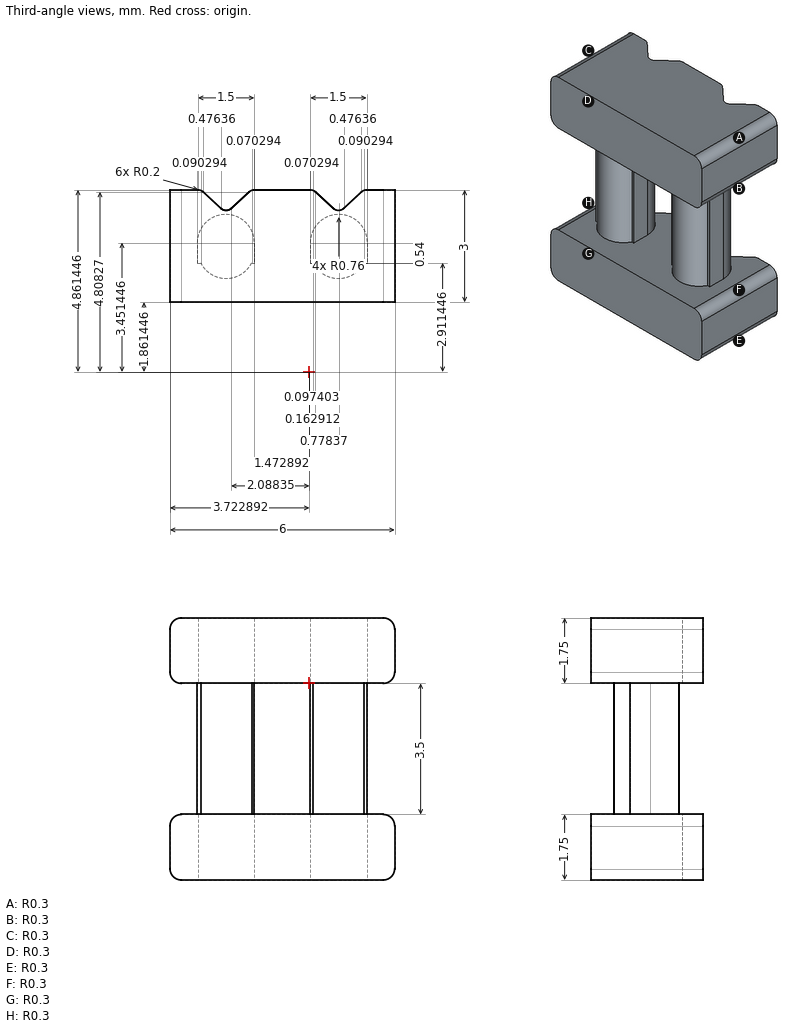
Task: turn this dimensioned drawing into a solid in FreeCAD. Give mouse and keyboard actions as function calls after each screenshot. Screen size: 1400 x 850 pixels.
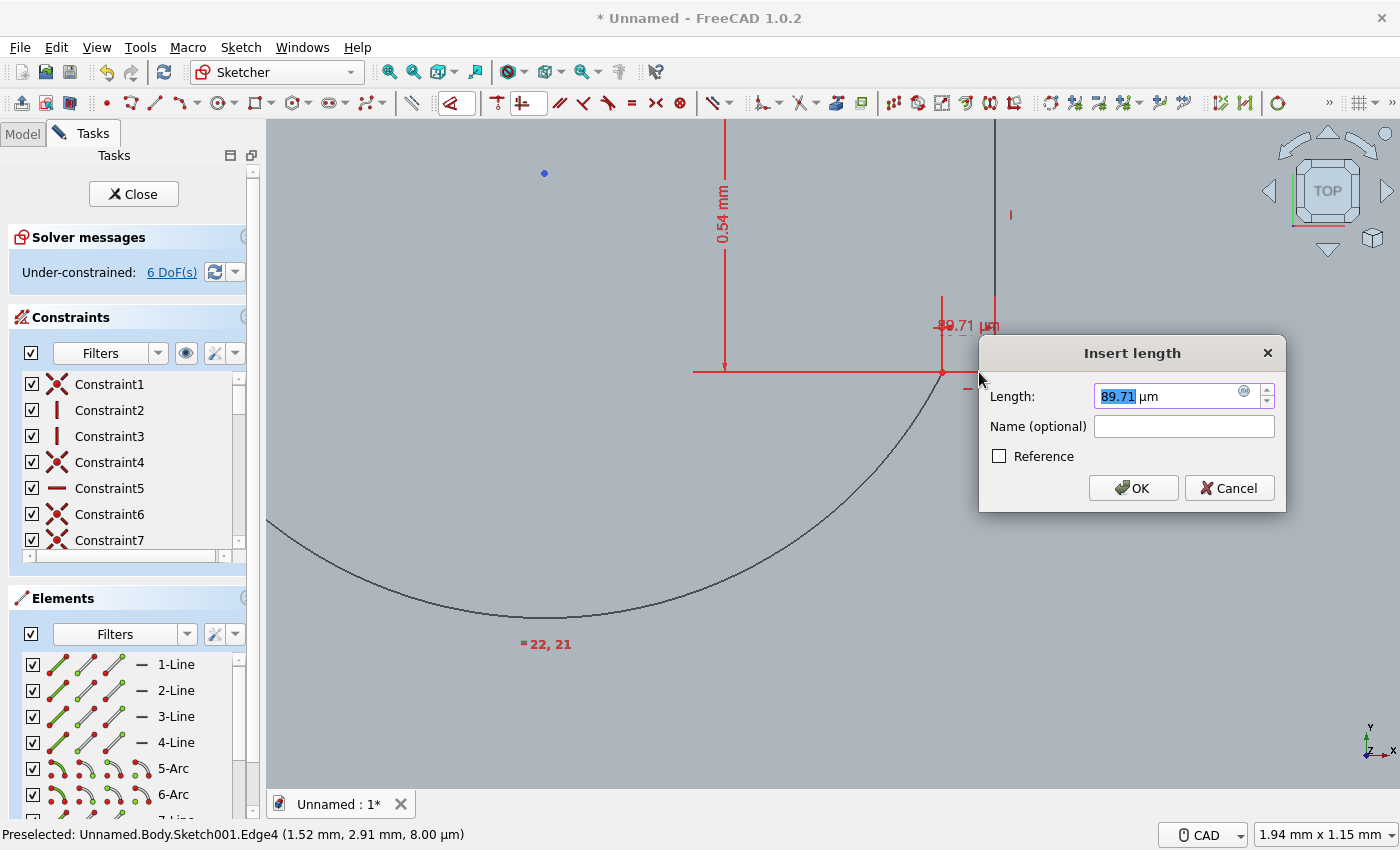
key(ctrl+a)
text(0.090294 mm)
key(Return)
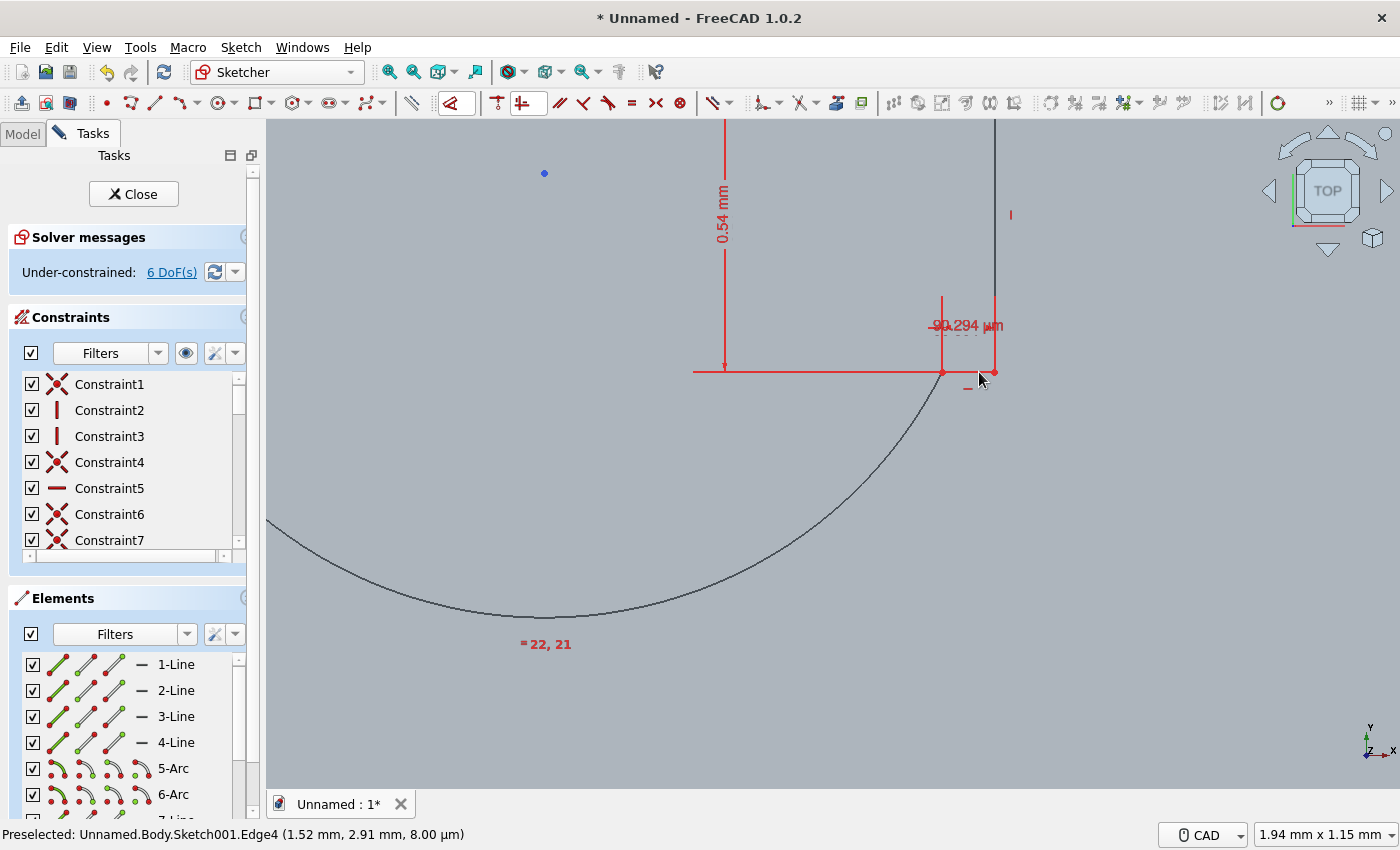
scroll(982, 377, down, 9)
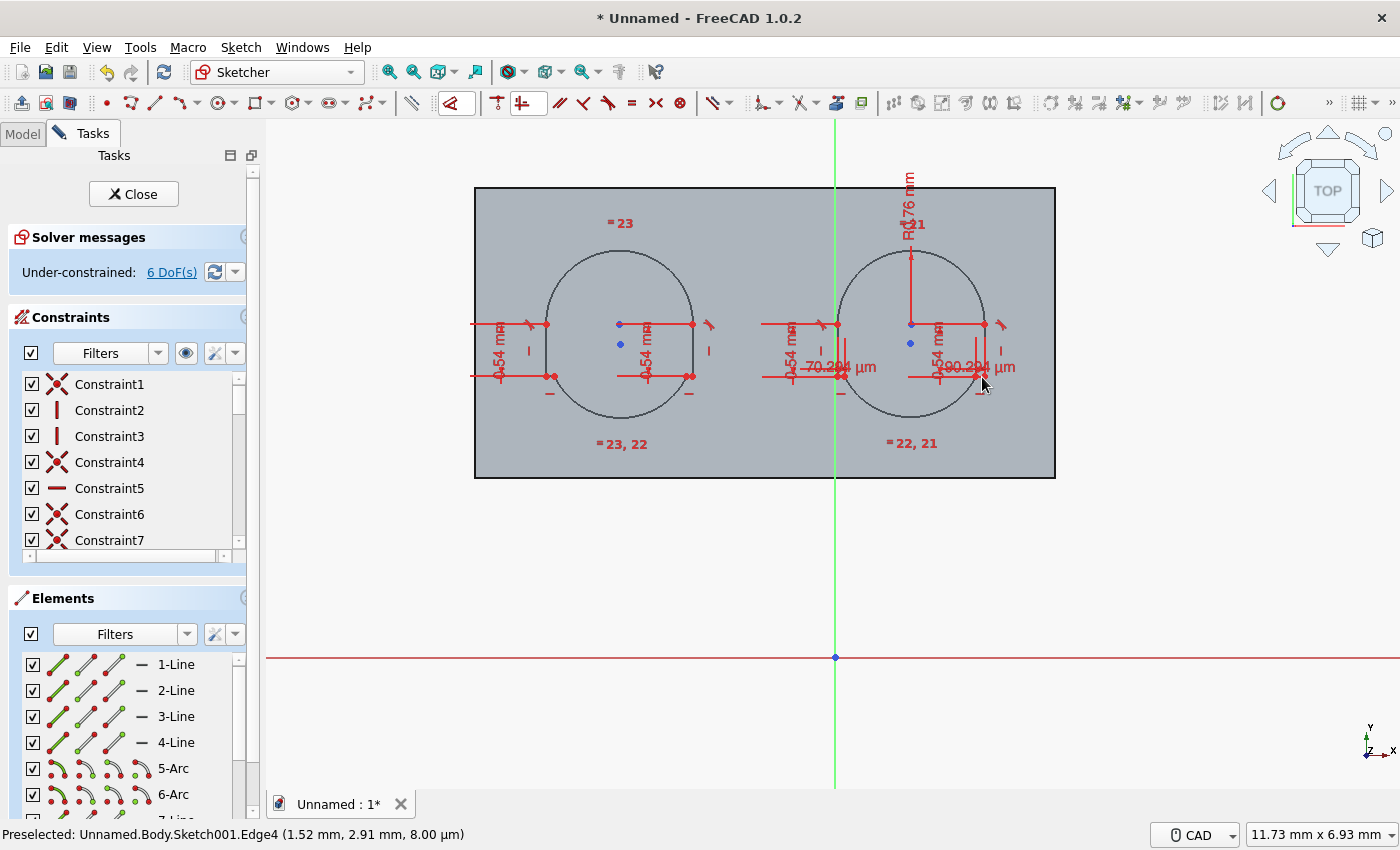
scroll(691, 376, up, 11)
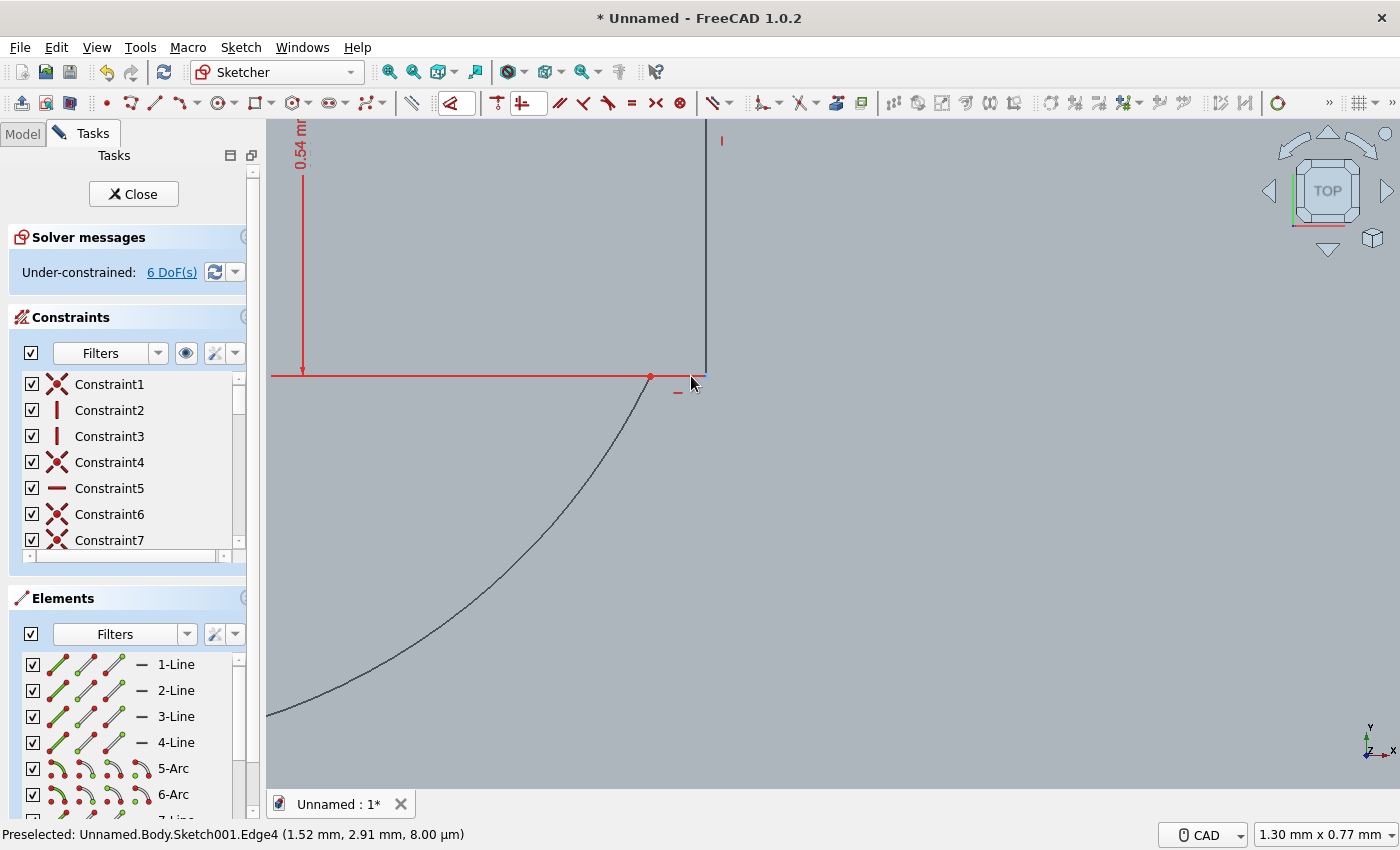
click(689, 376)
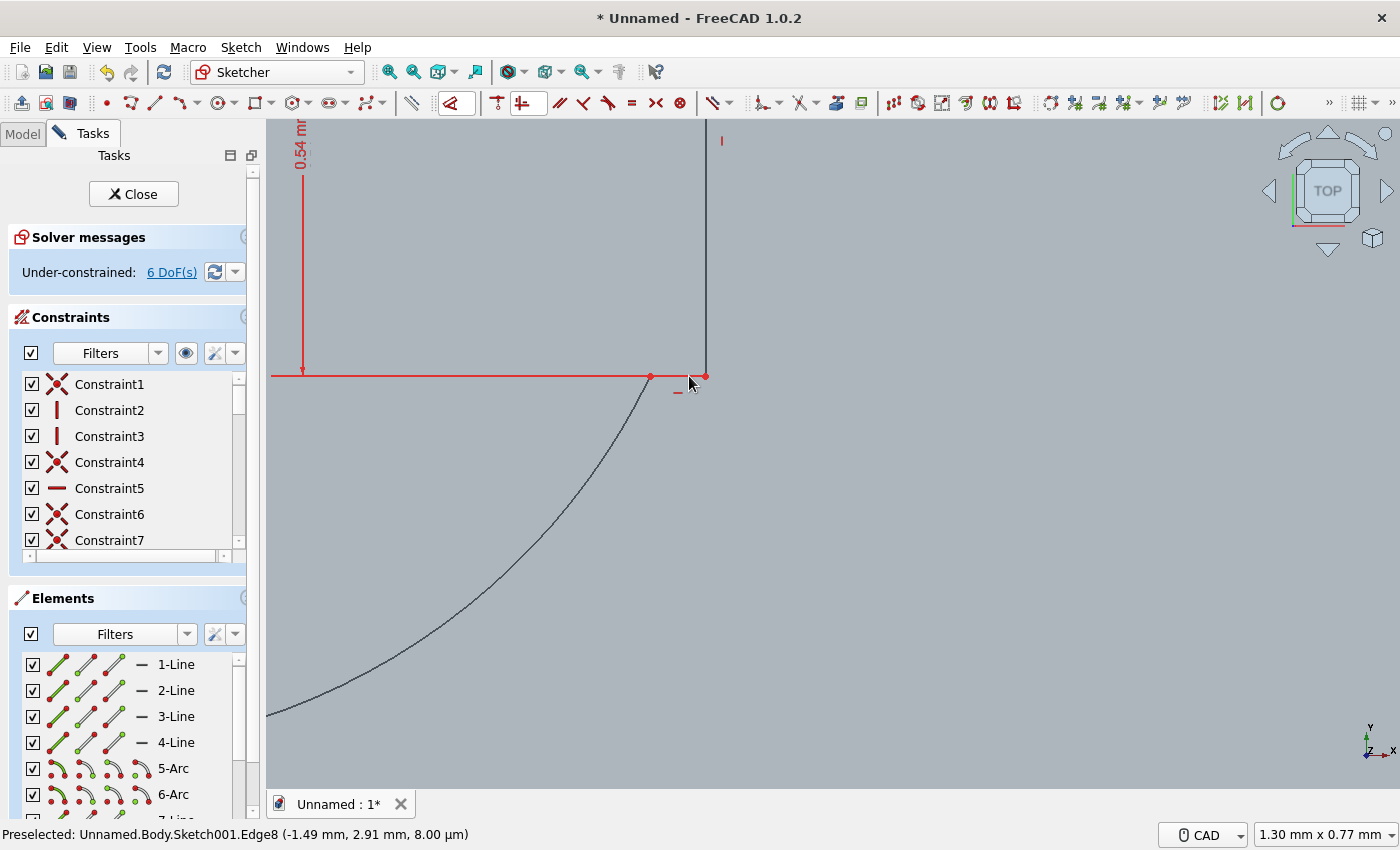
key(l)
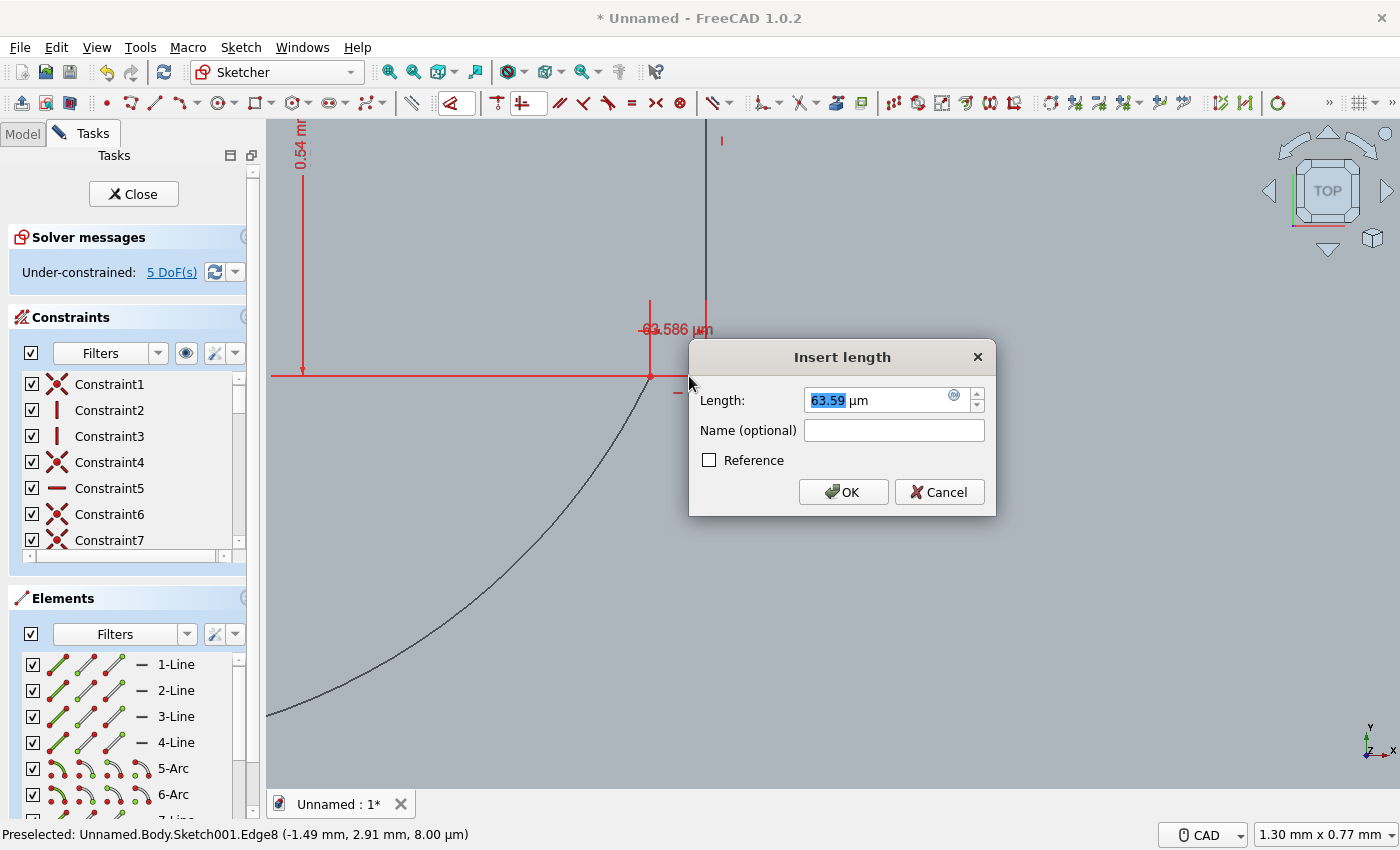
key(ctrl+a)
text(0.070294 mm)
key(Return)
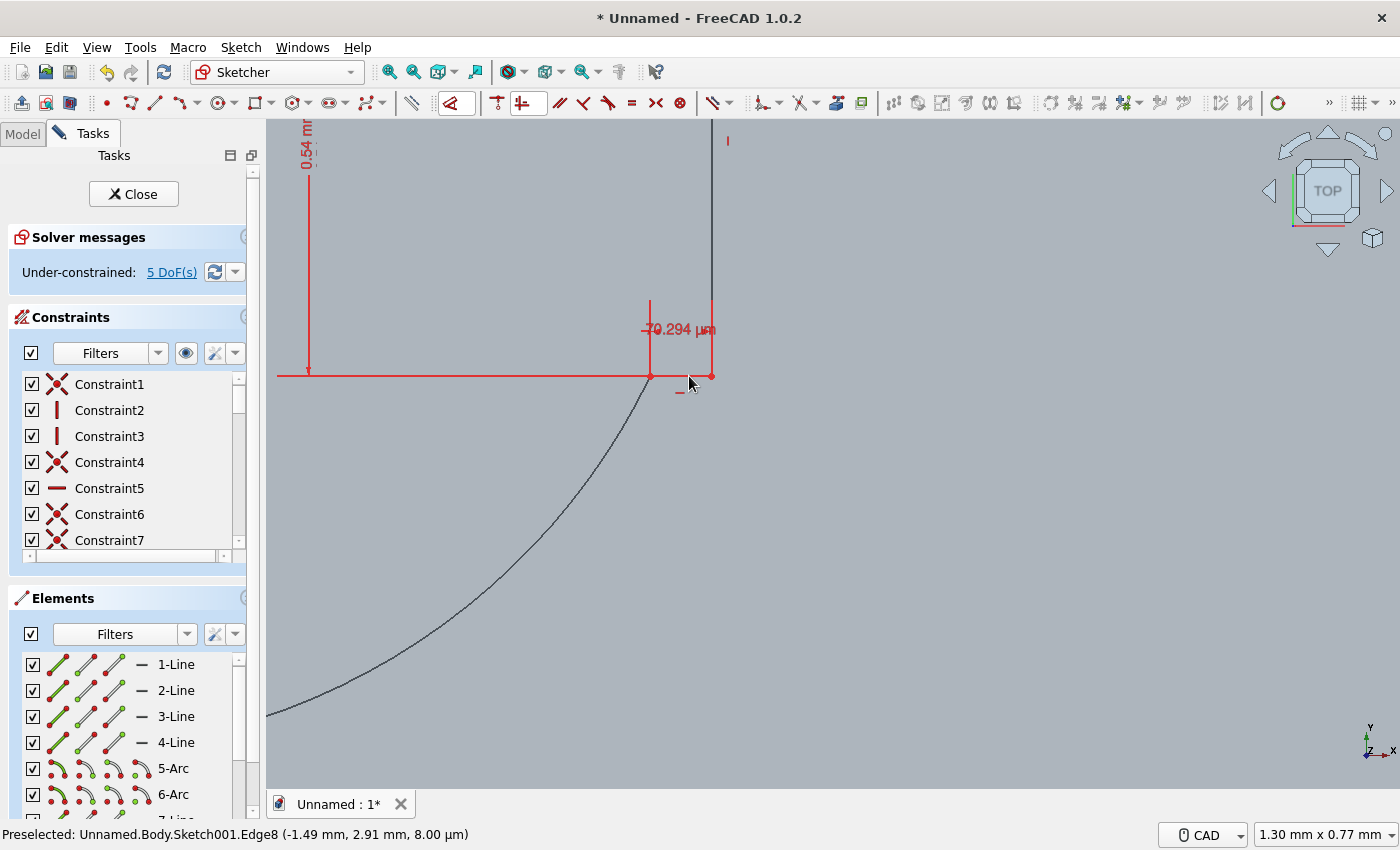
scroll(691, 376, down, 11)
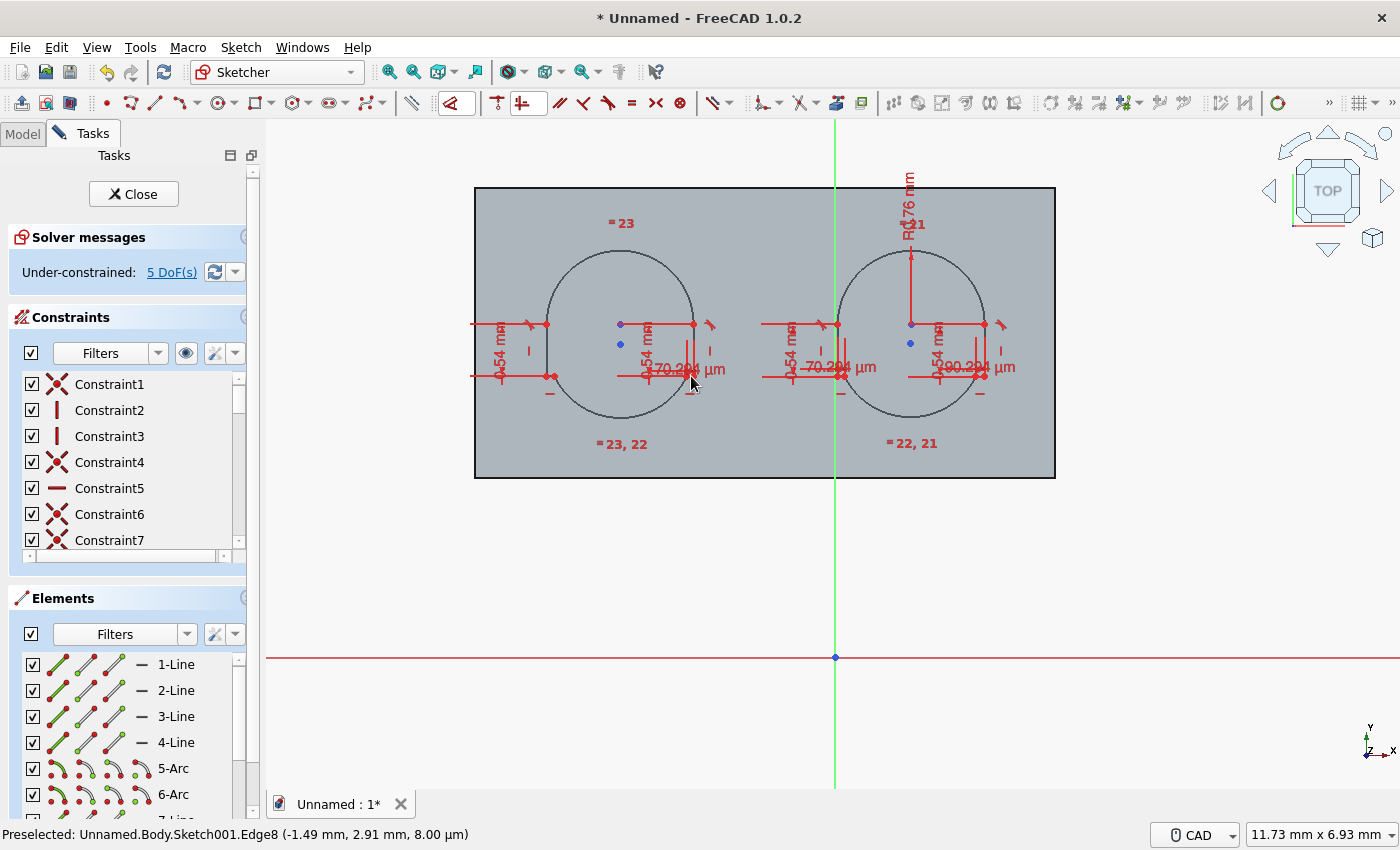
scroll(552, 376, up, 9)